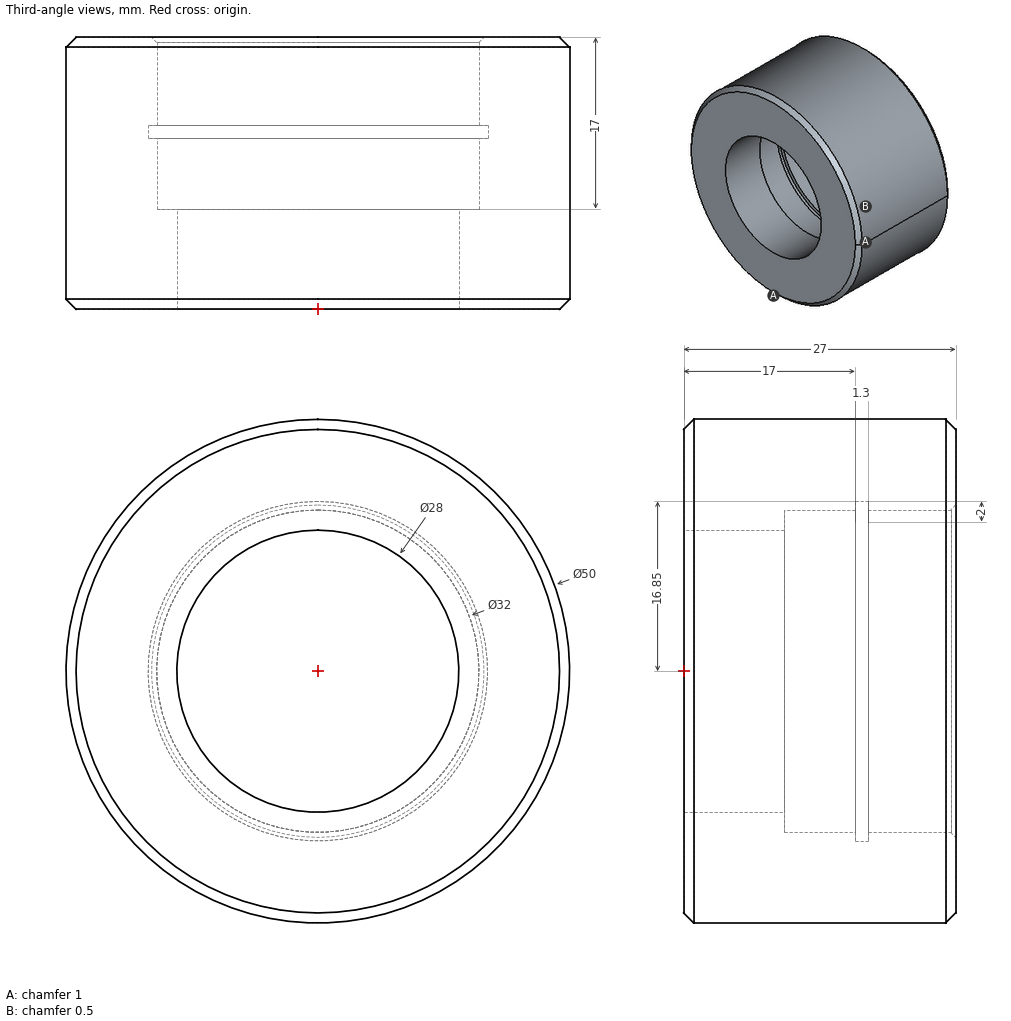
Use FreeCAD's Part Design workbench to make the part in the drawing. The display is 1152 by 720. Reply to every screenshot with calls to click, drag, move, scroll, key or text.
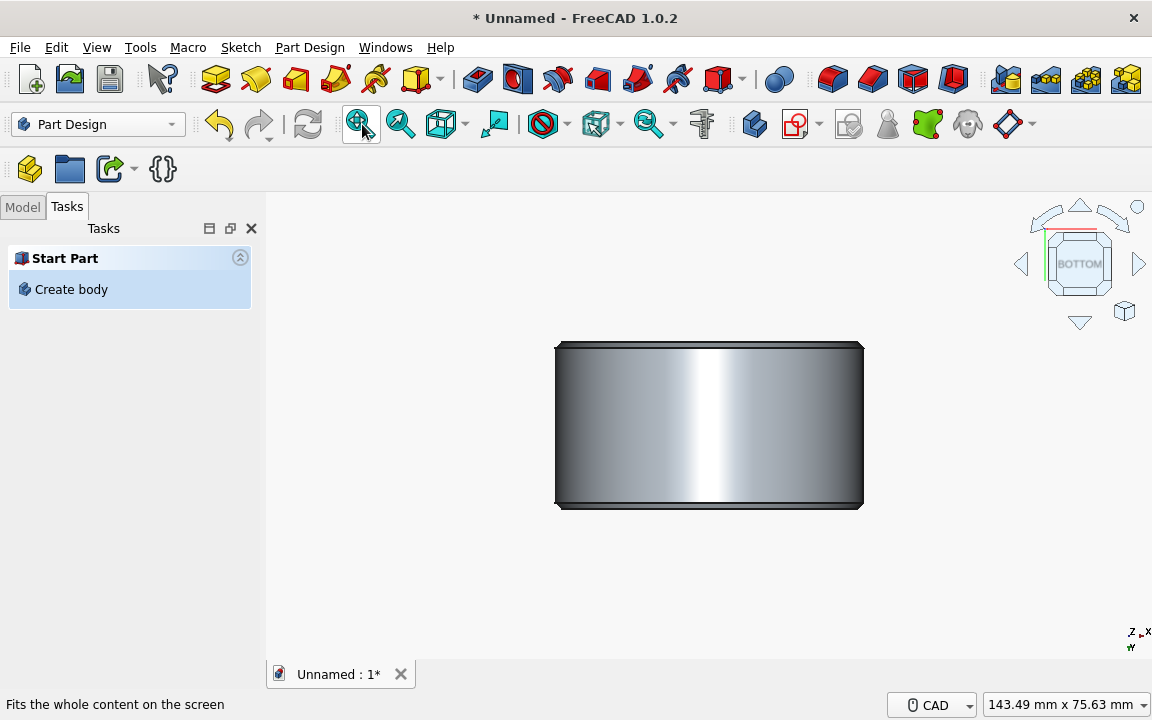
key(4)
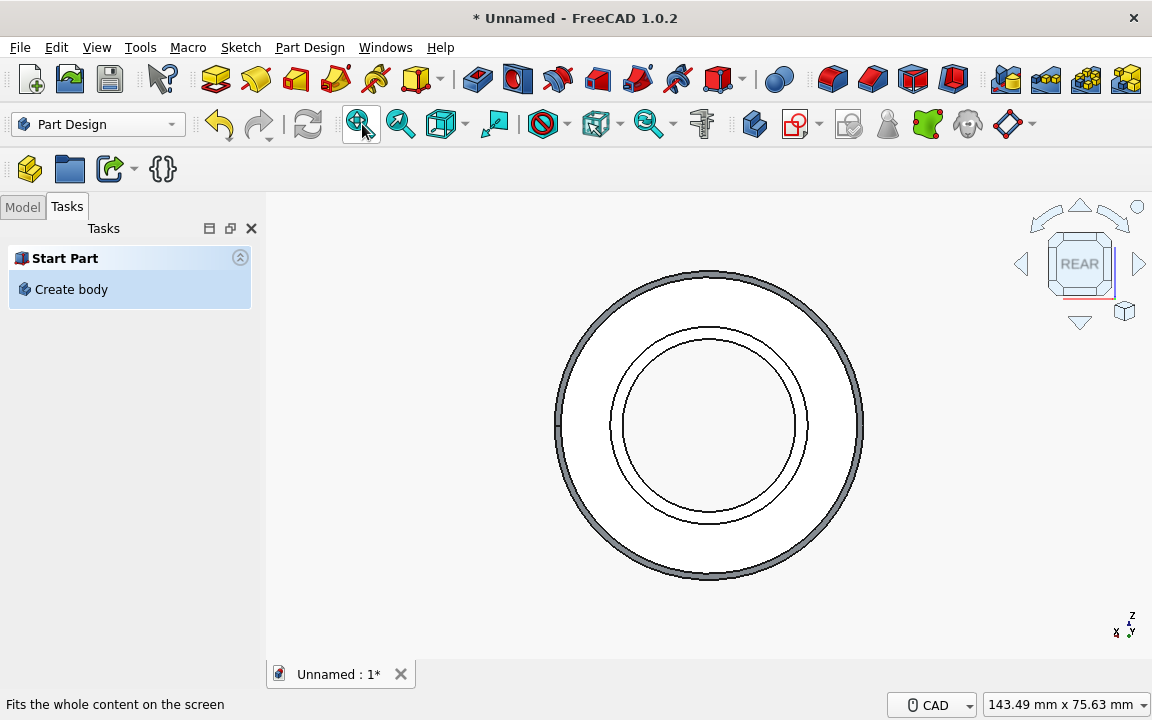
click(789, 366)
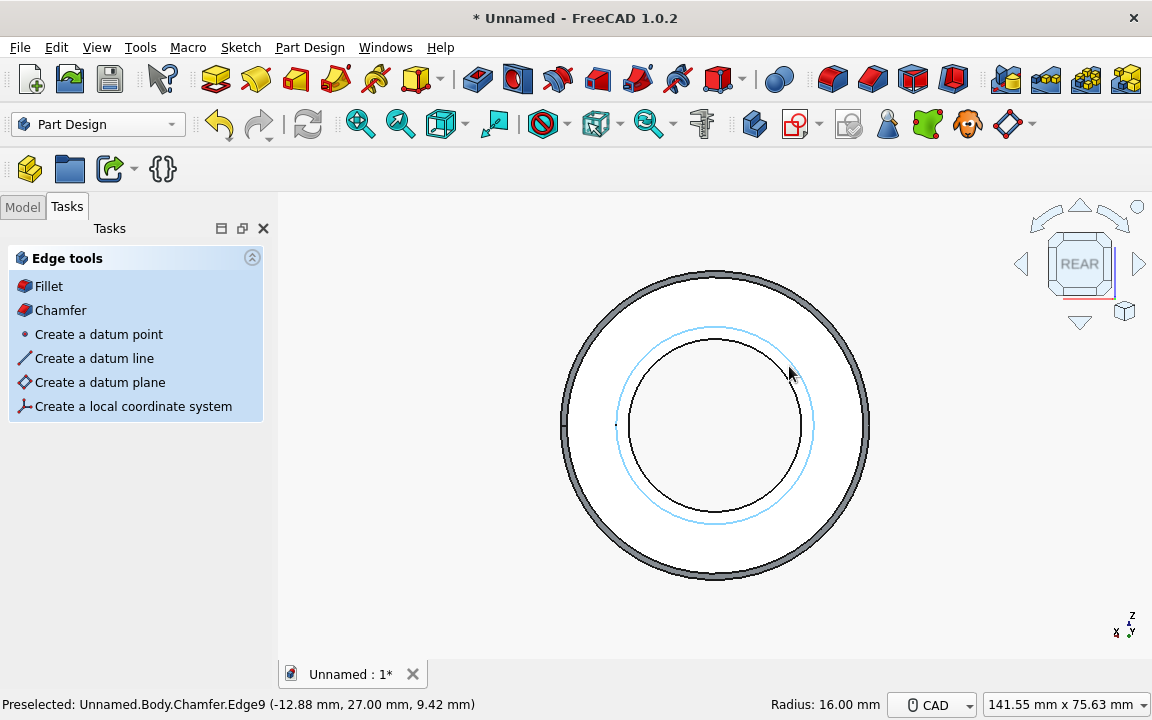
click(874, 80)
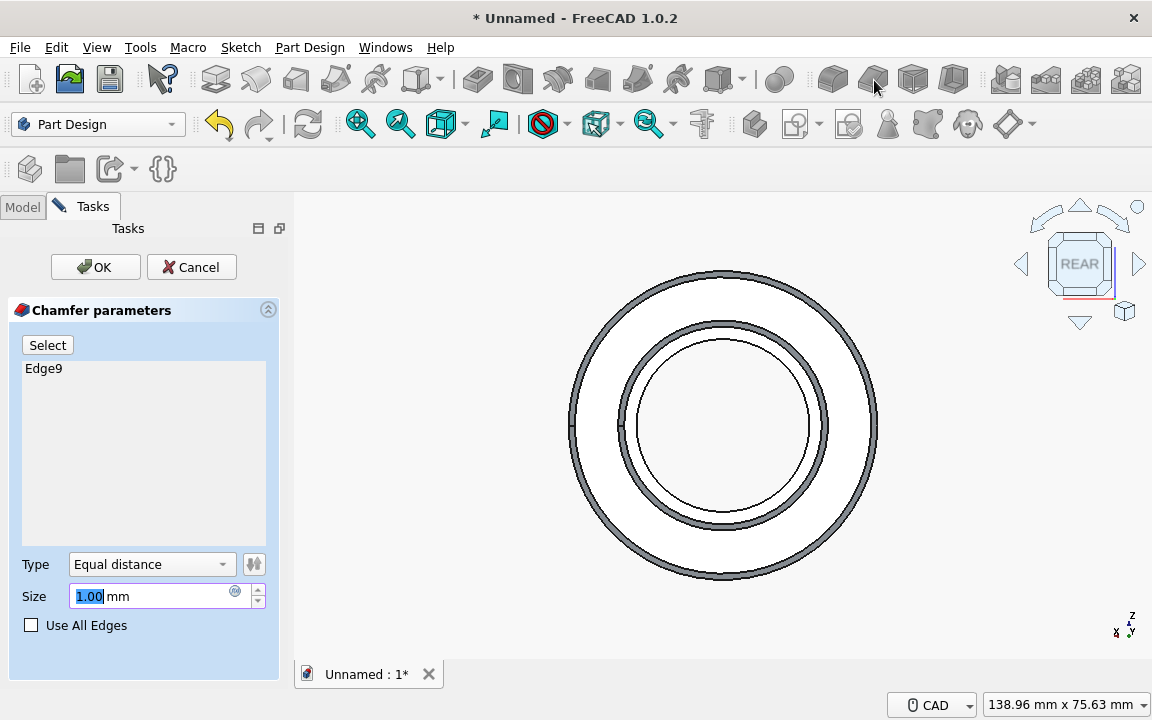
text(0.5)
key(Tab)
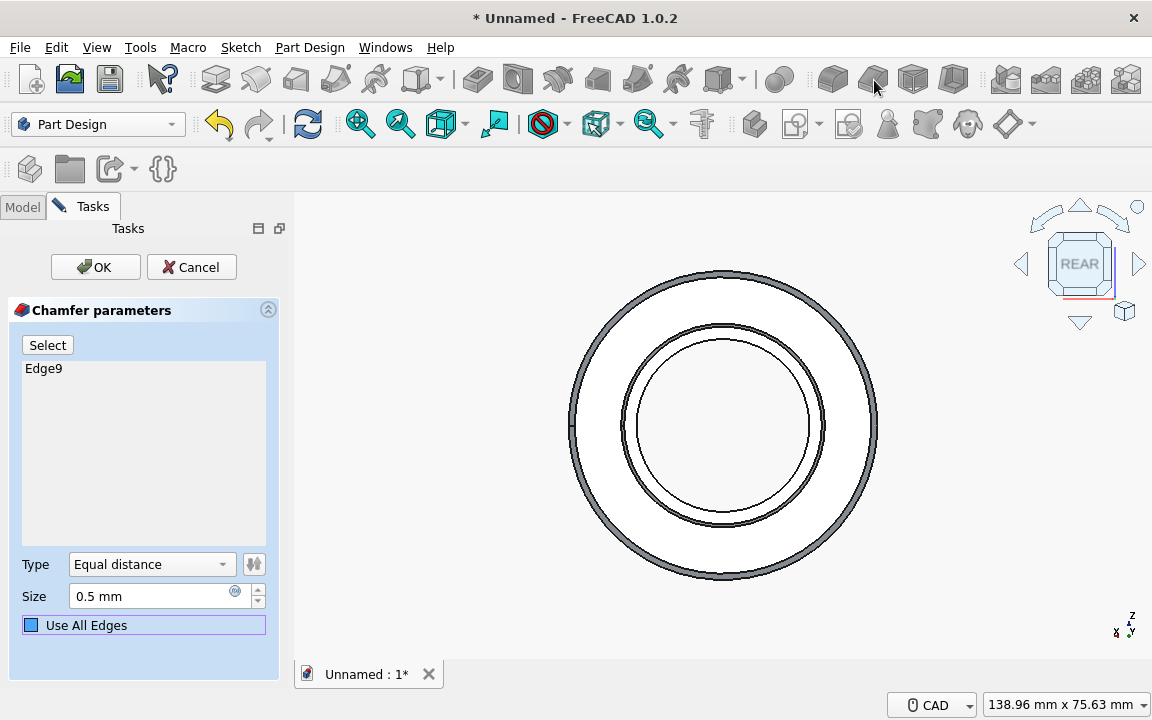
click(96, 267)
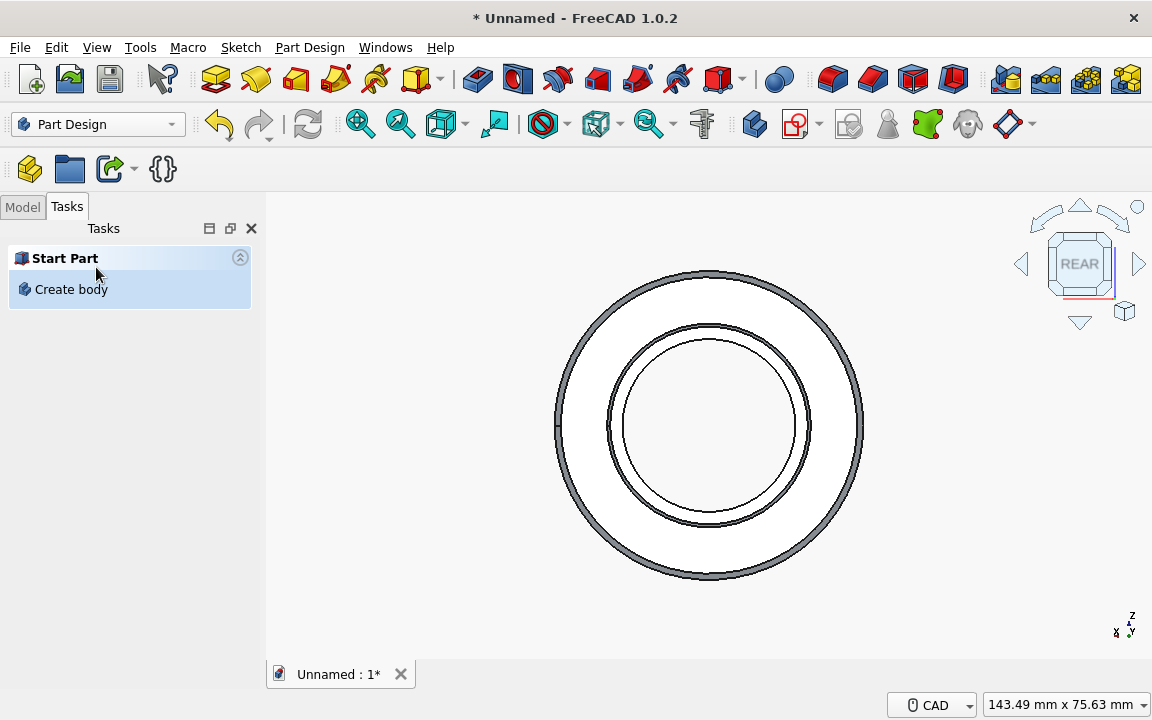
click(796, 124)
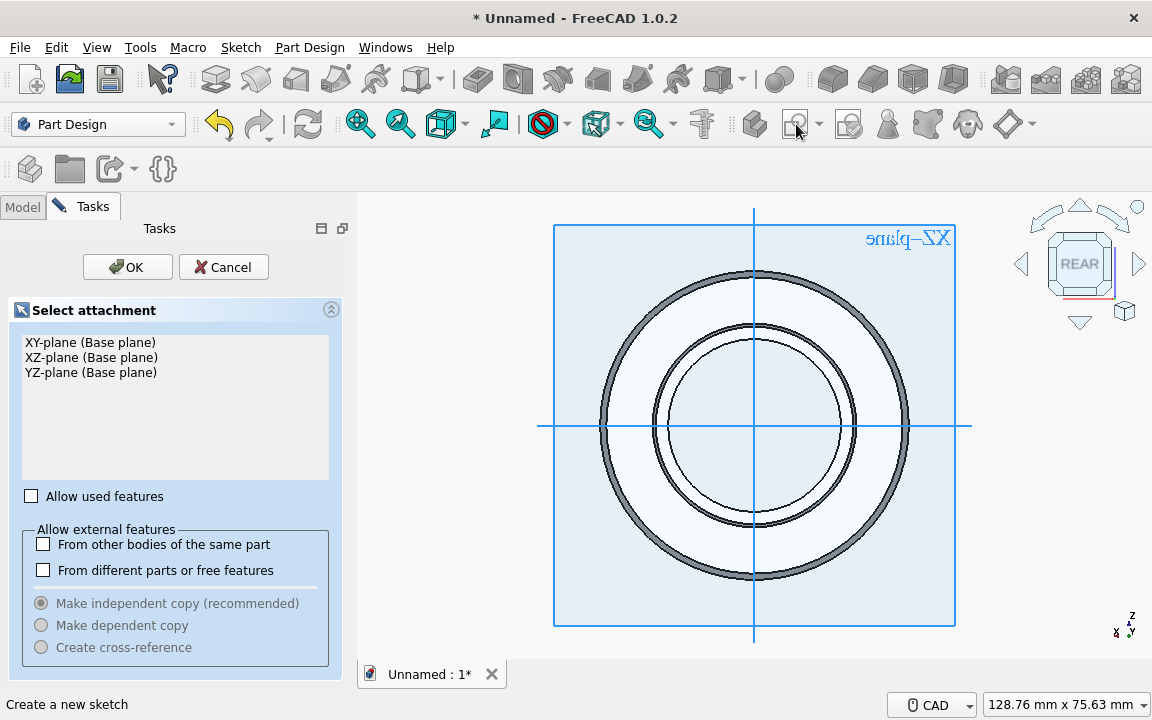
click(82, 372)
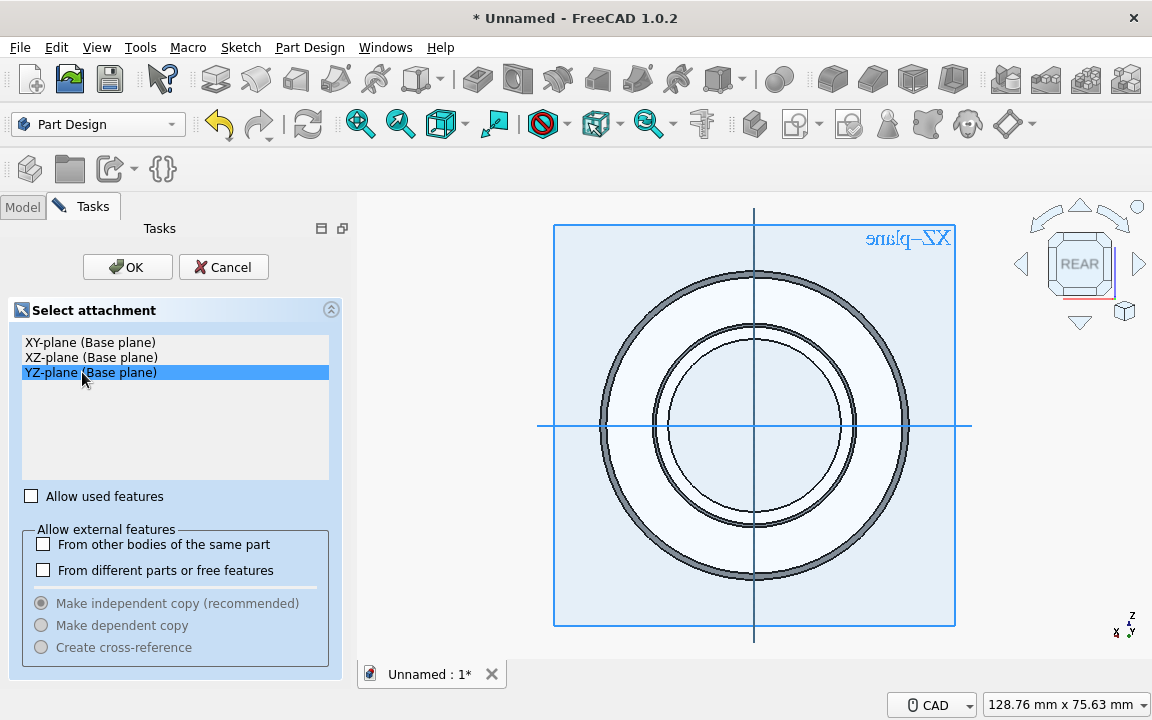
click(128, 267)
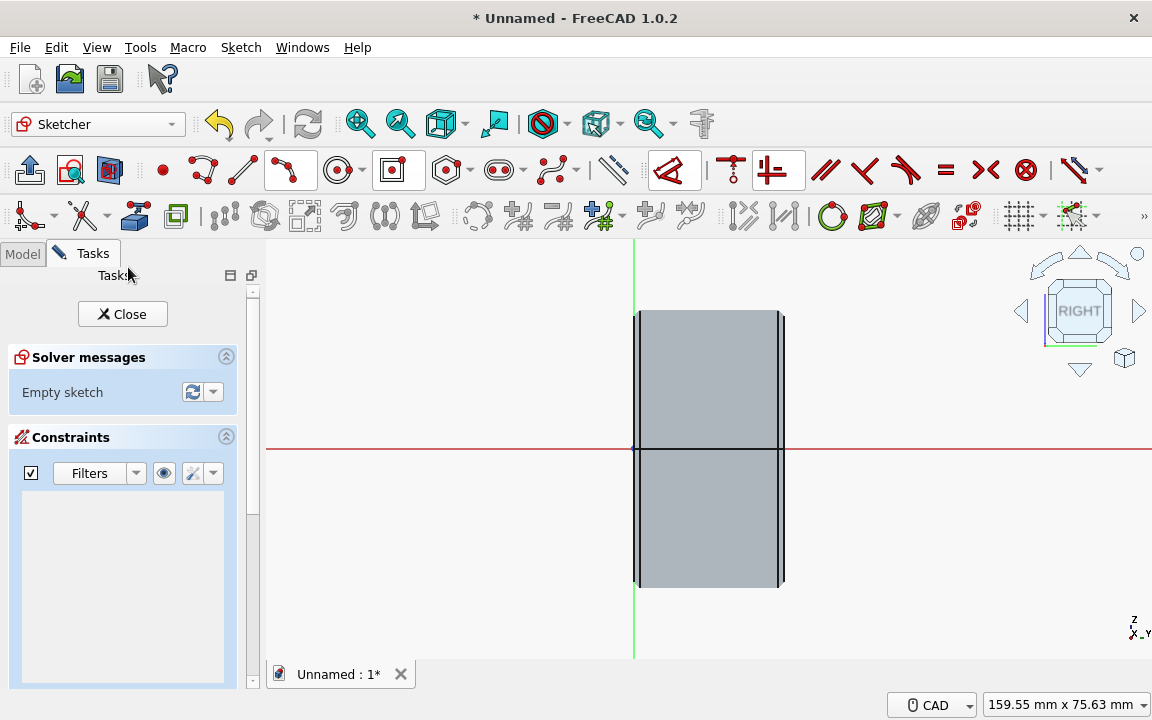
click(110, 170)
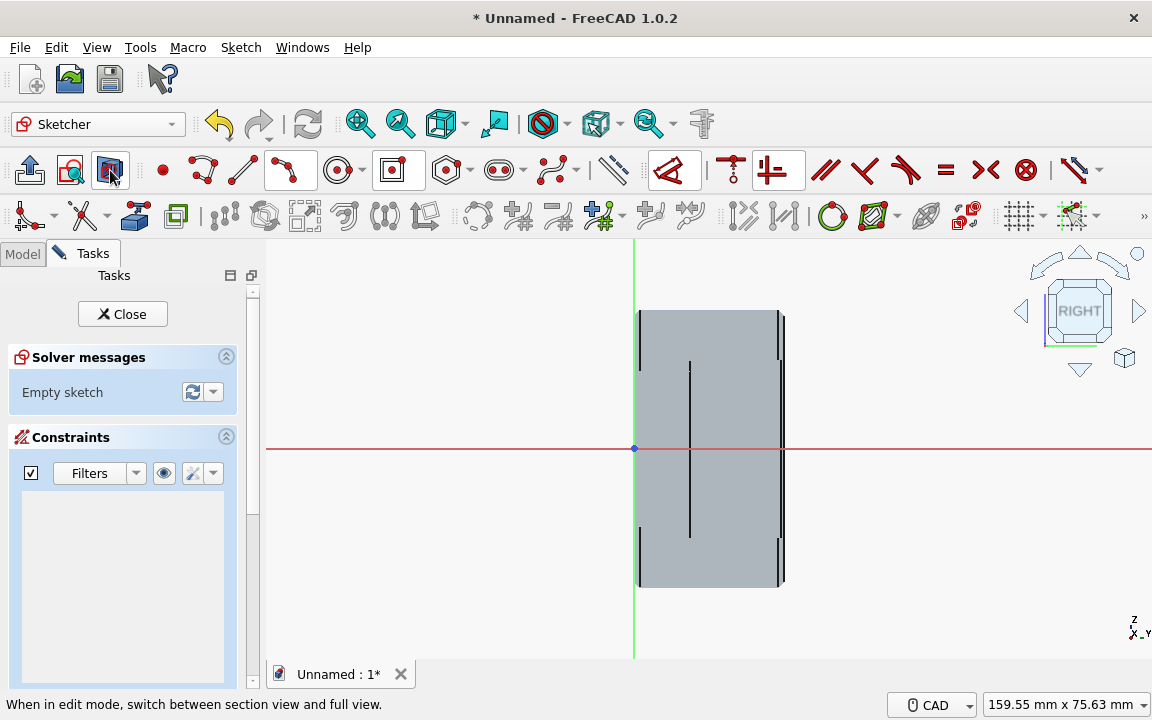
scroll(737, 356, up, 15)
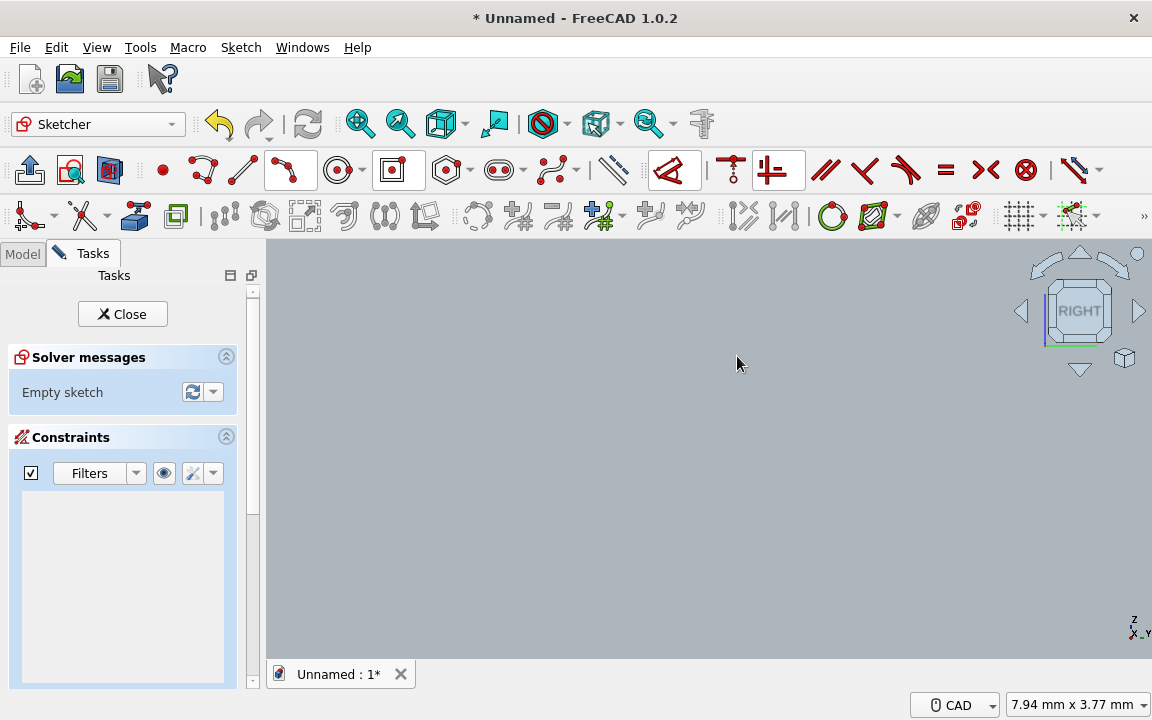
click(420, 170)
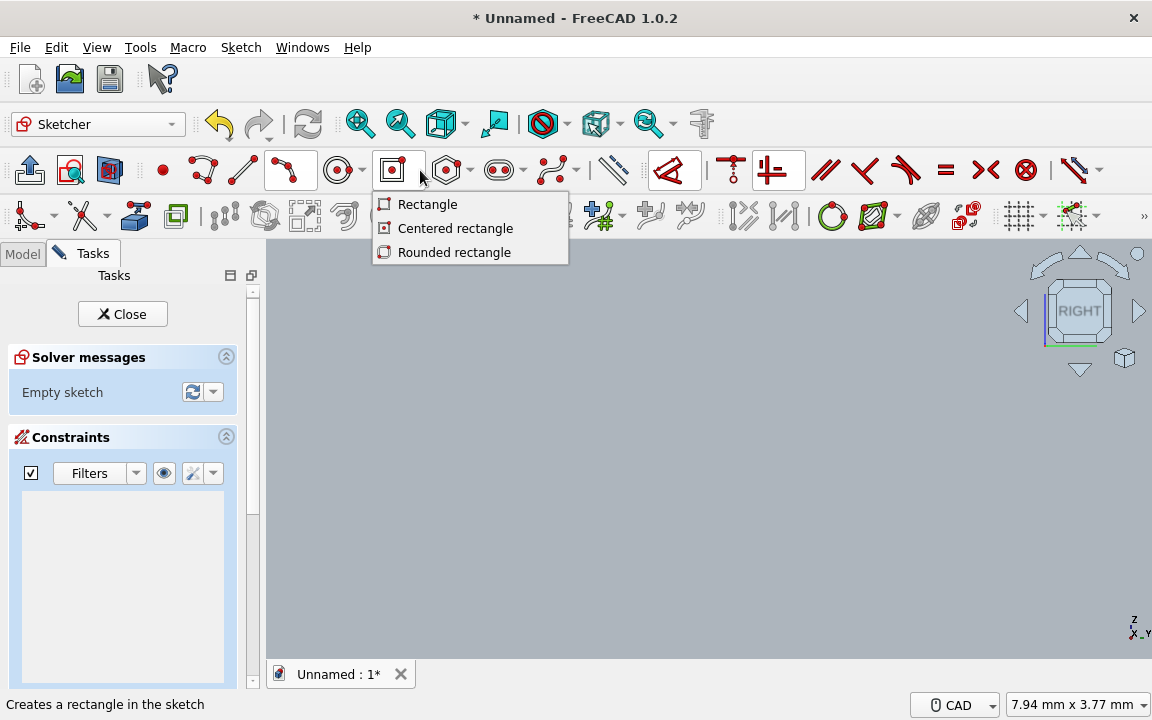
click(470, 204)